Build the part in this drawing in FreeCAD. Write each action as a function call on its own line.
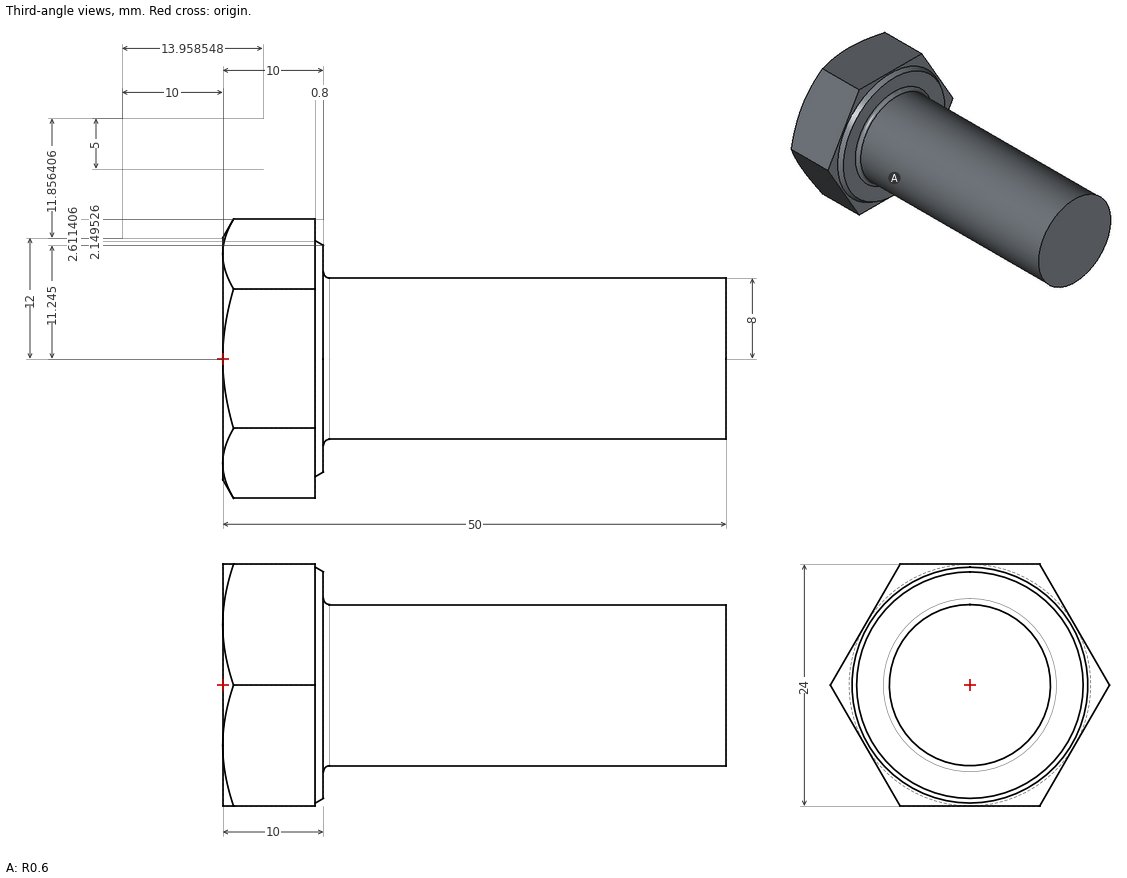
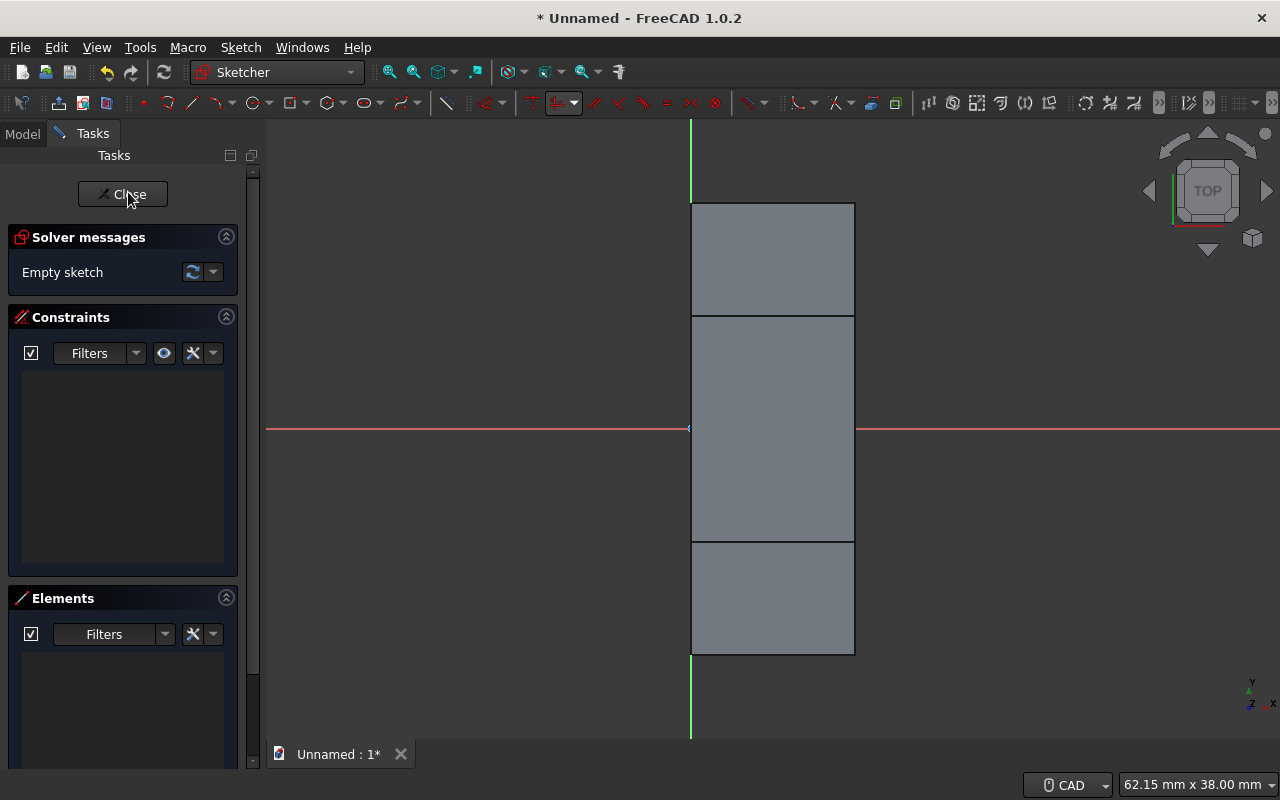
click(108, 104)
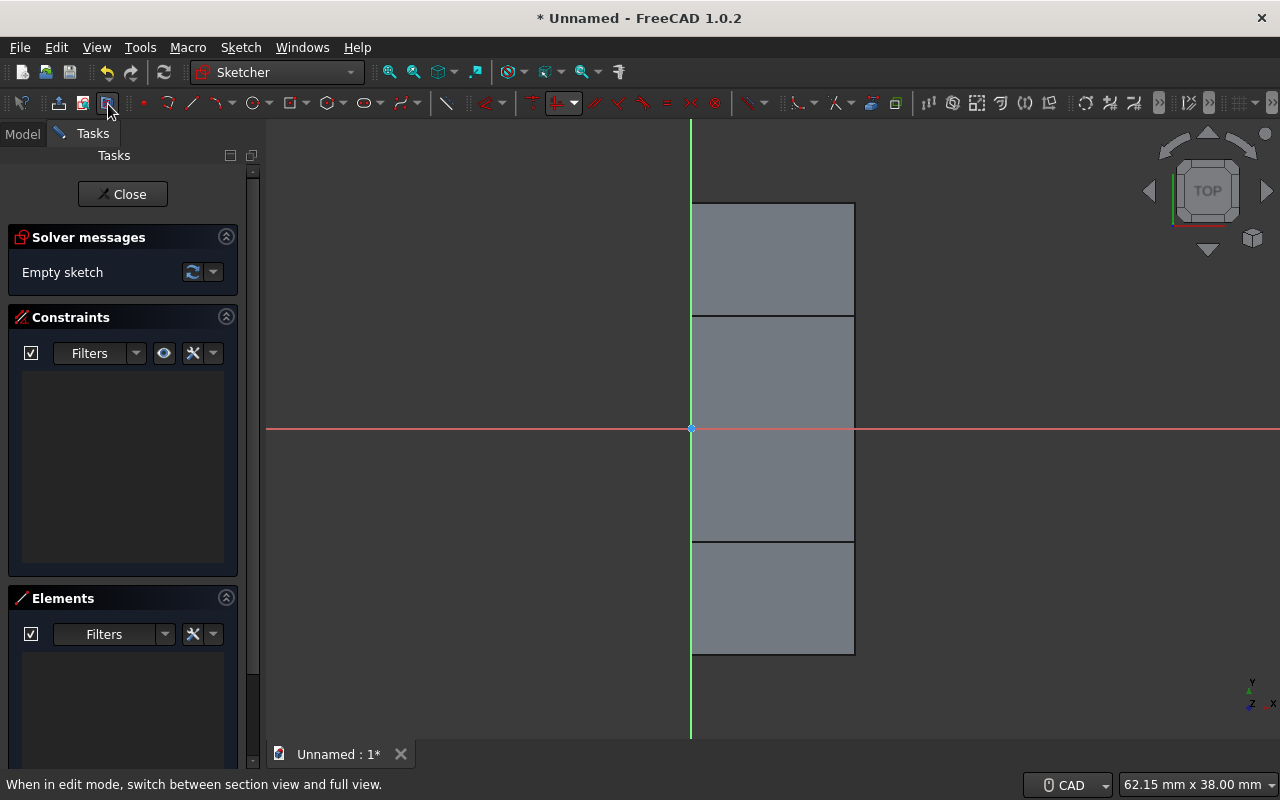
scroll(294, 508, down, 3)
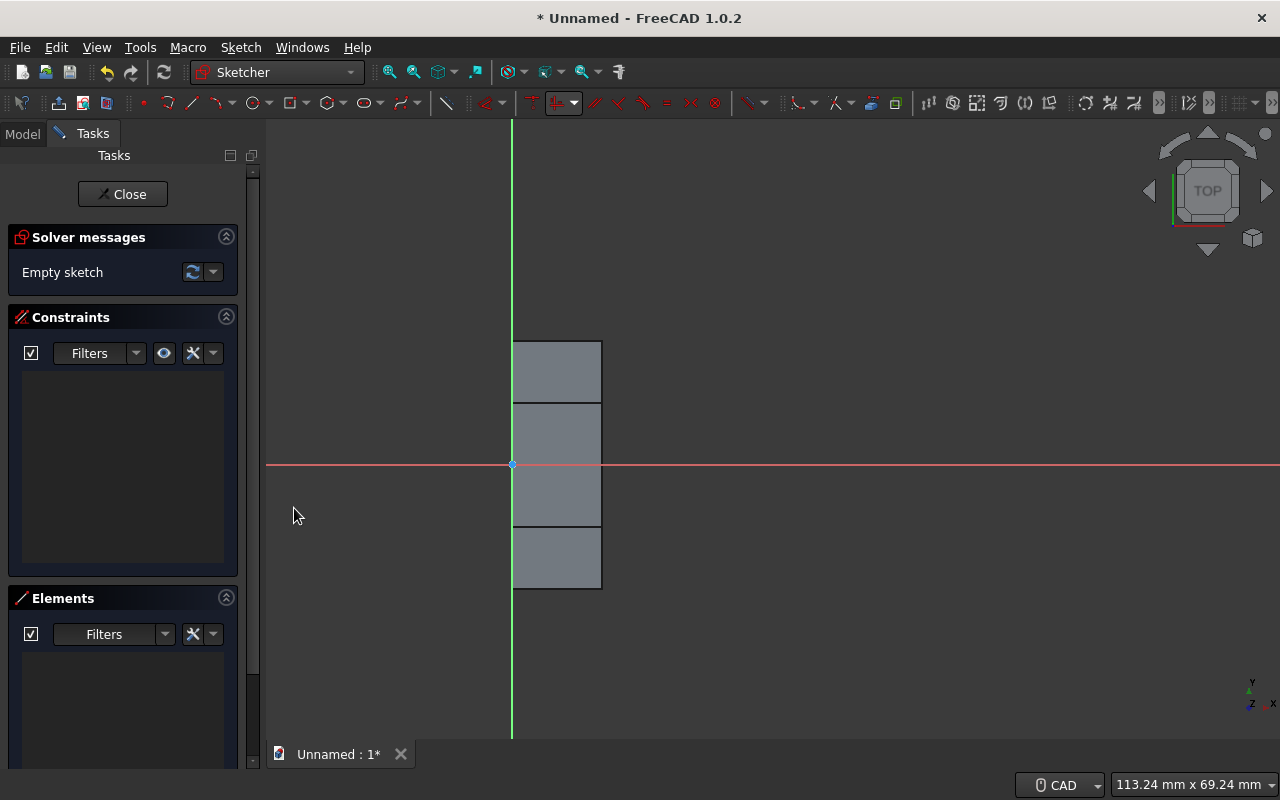
click(308, 104)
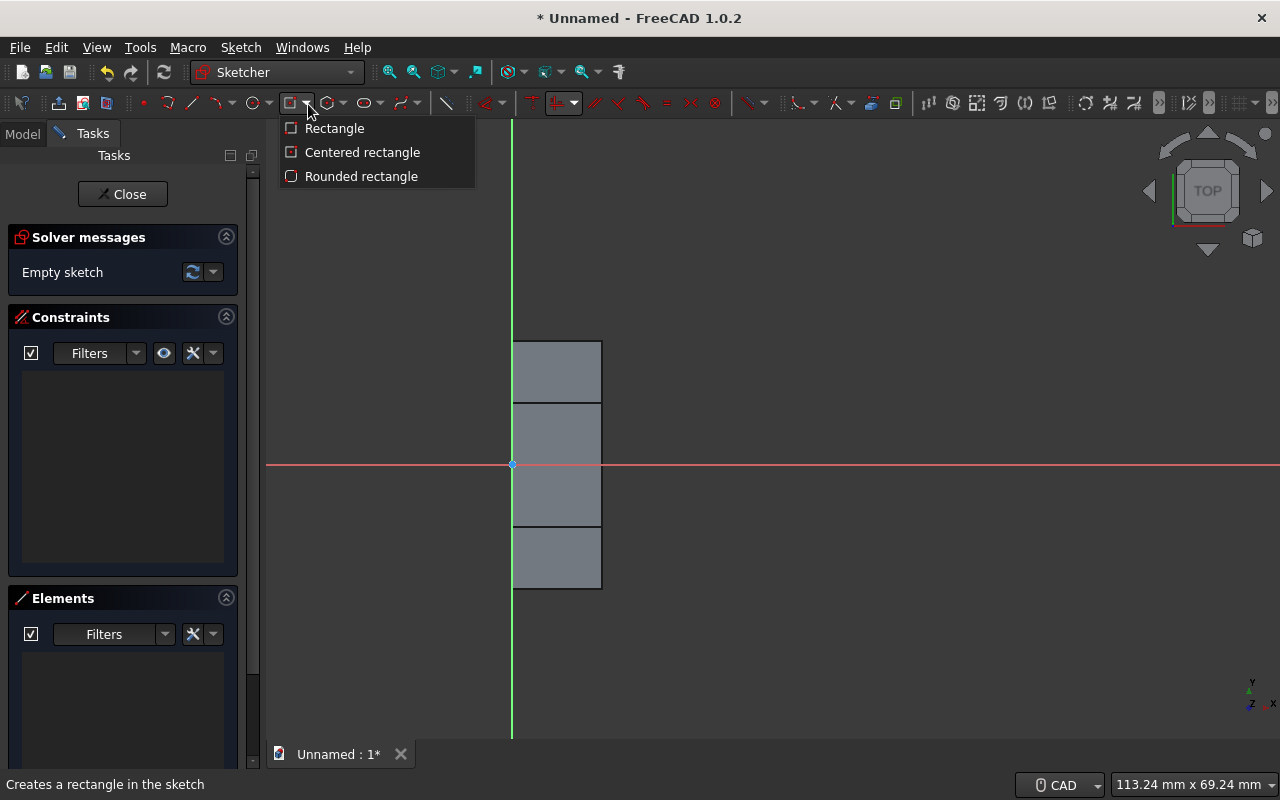
click(378, 128)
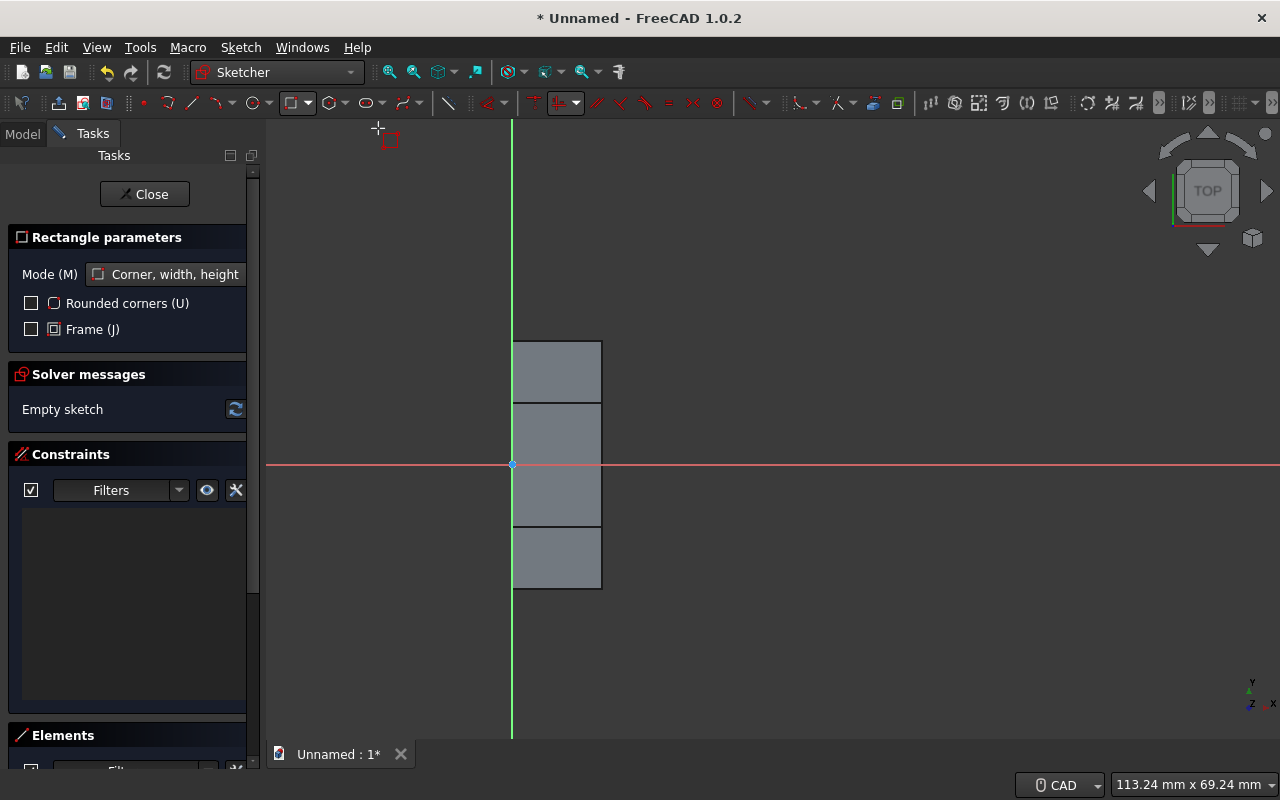
click(512, 465)
move(960, 393)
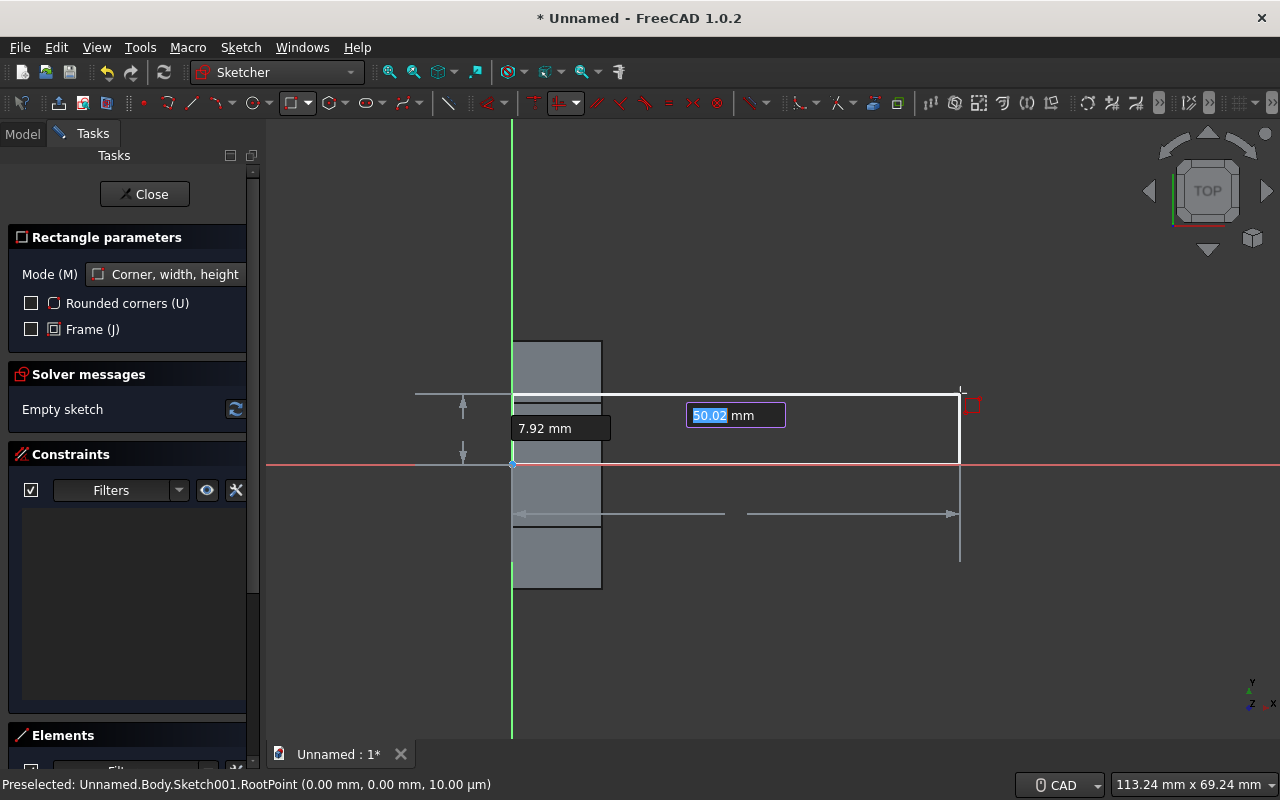
text(50)
key(Tab)
text(8)
key(Return)
key(Escape)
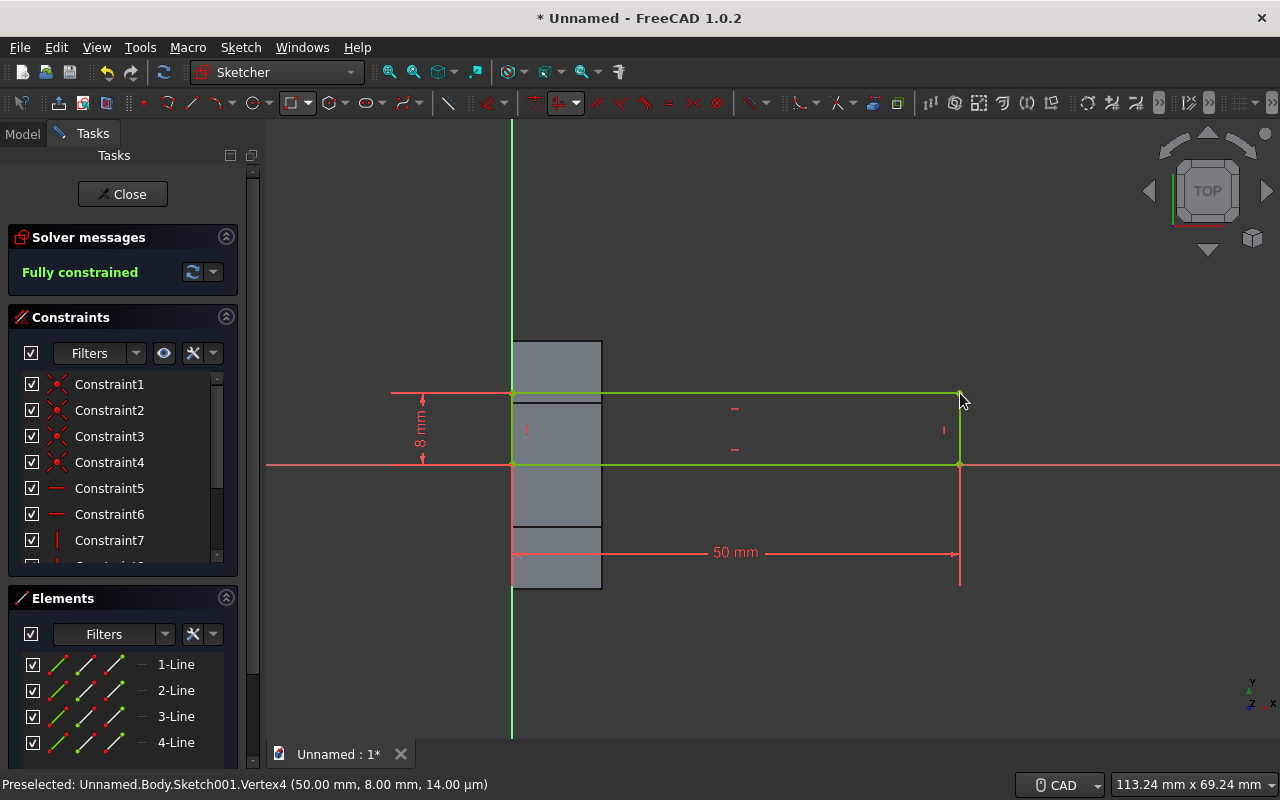
click(123, 194)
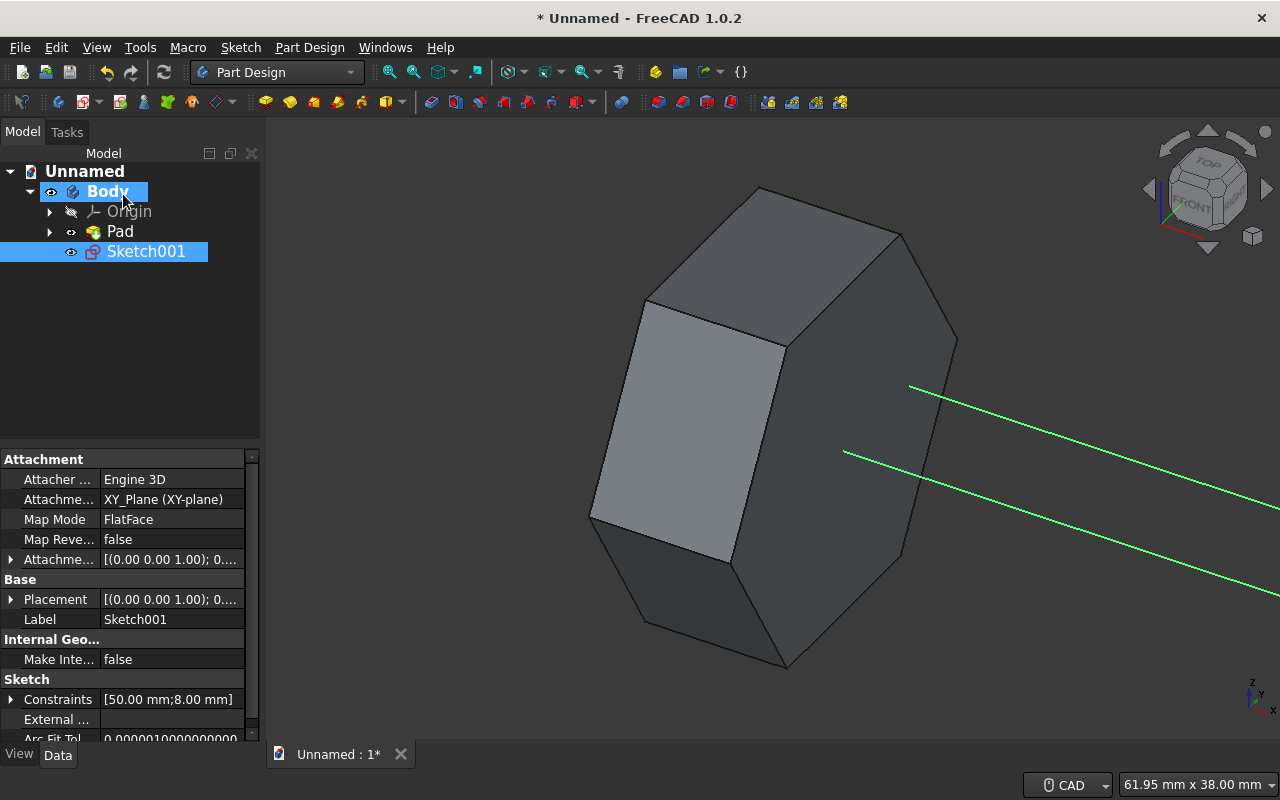
click(290, 102)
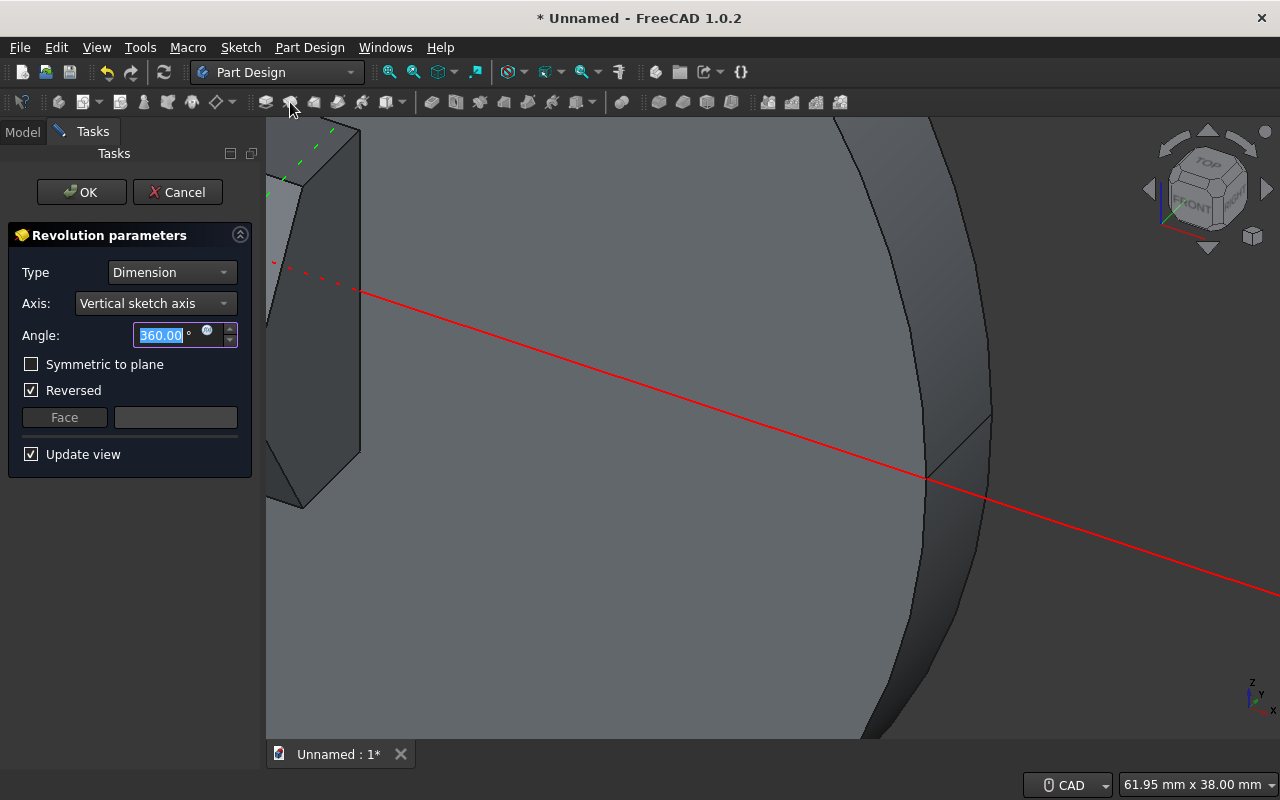
click(156, 304)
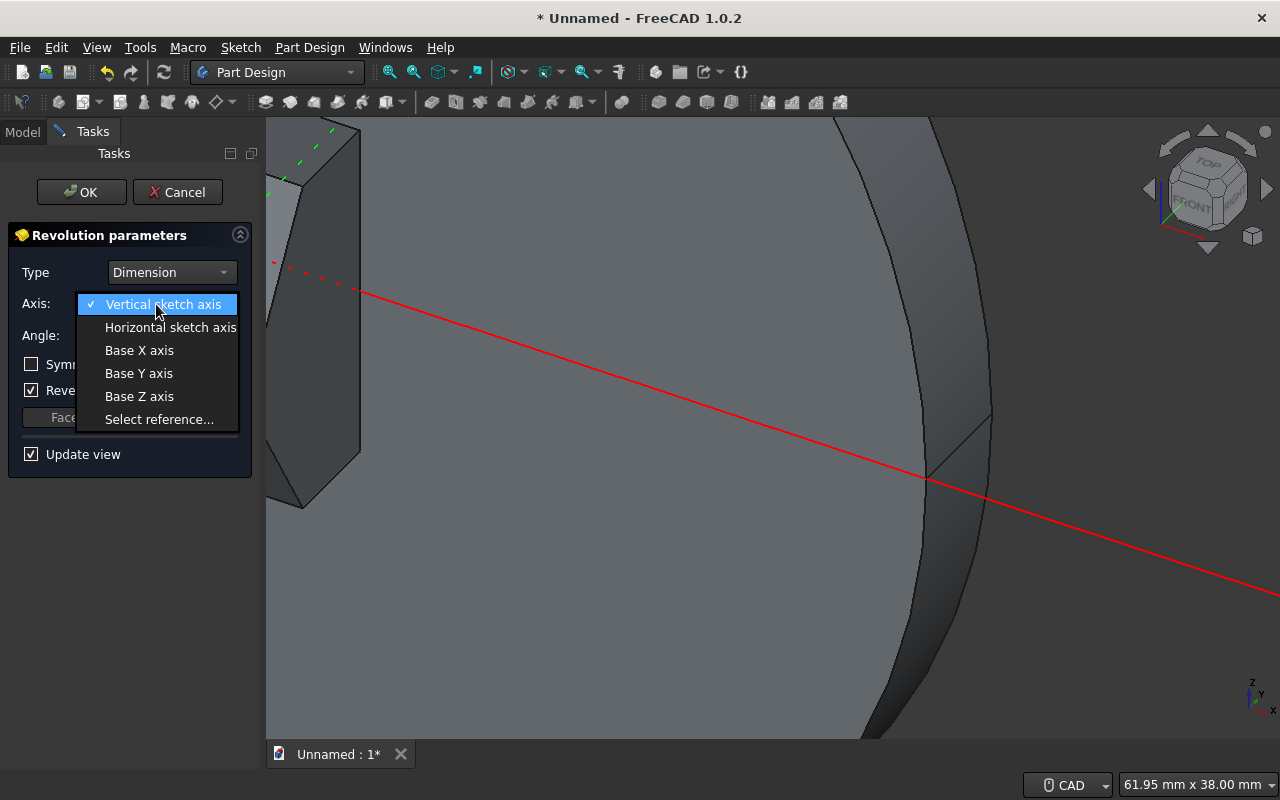
click(156, 328)